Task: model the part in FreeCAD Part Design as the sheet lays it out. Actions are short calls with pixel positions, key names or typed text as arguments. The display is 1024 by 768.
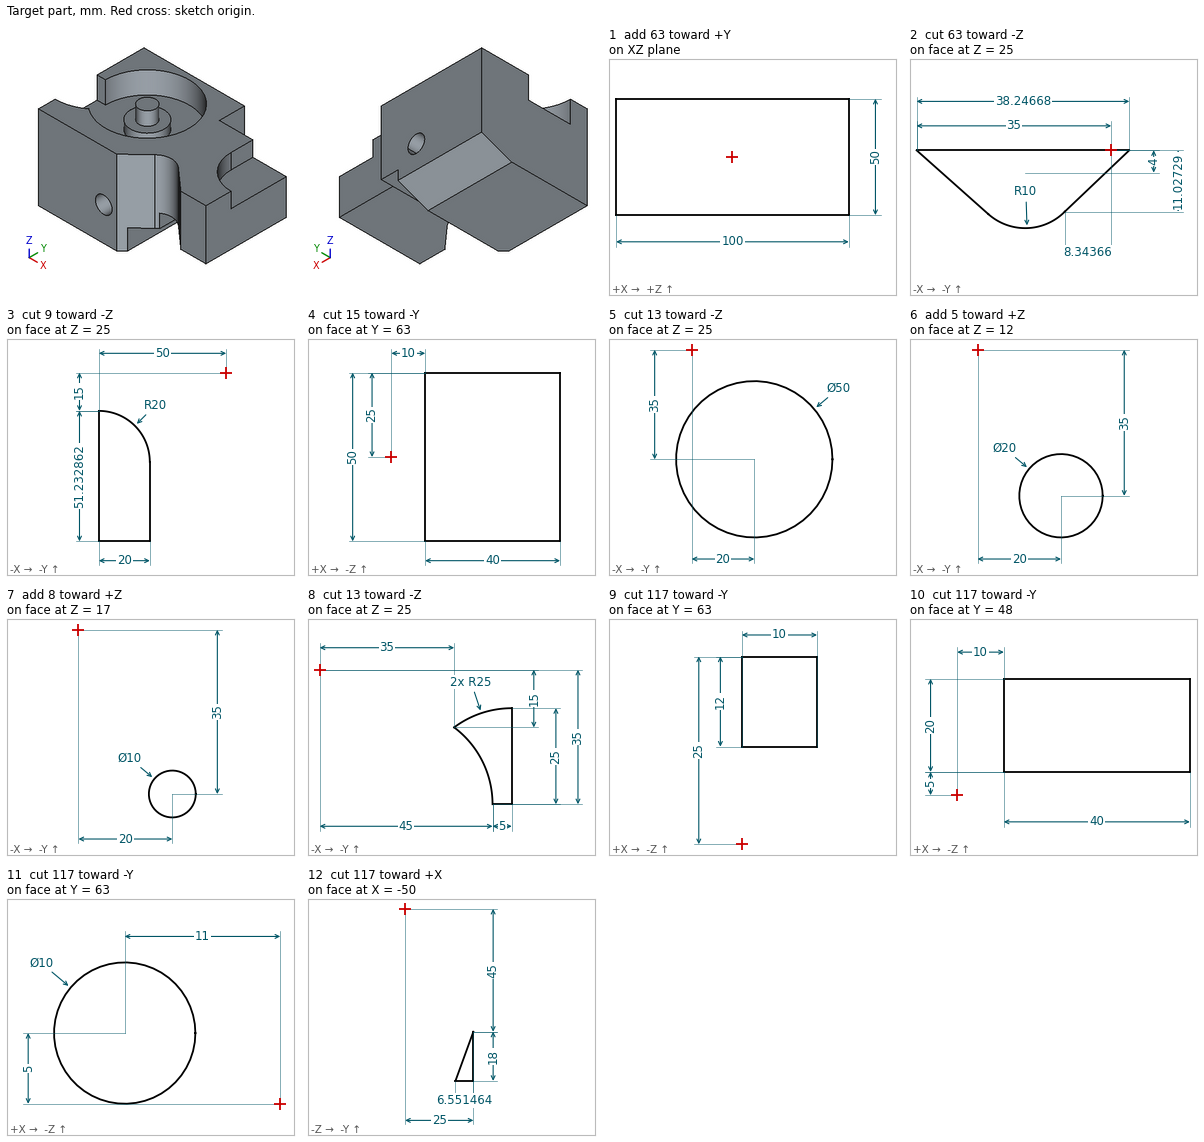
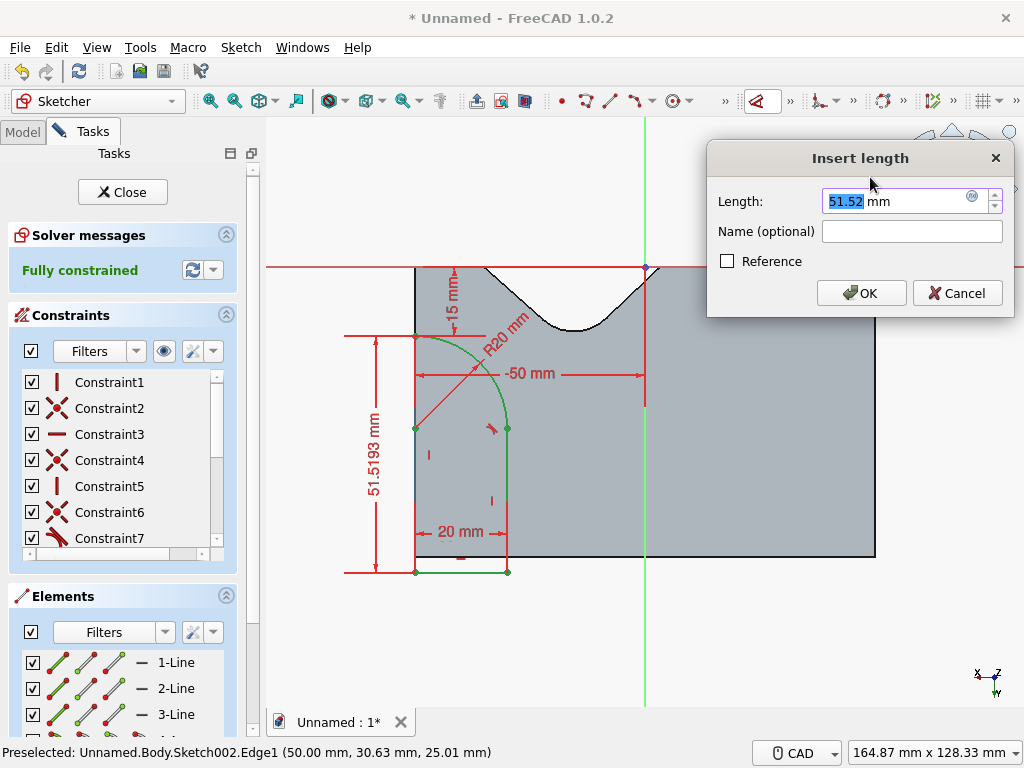
text(51.232862)
key(Return)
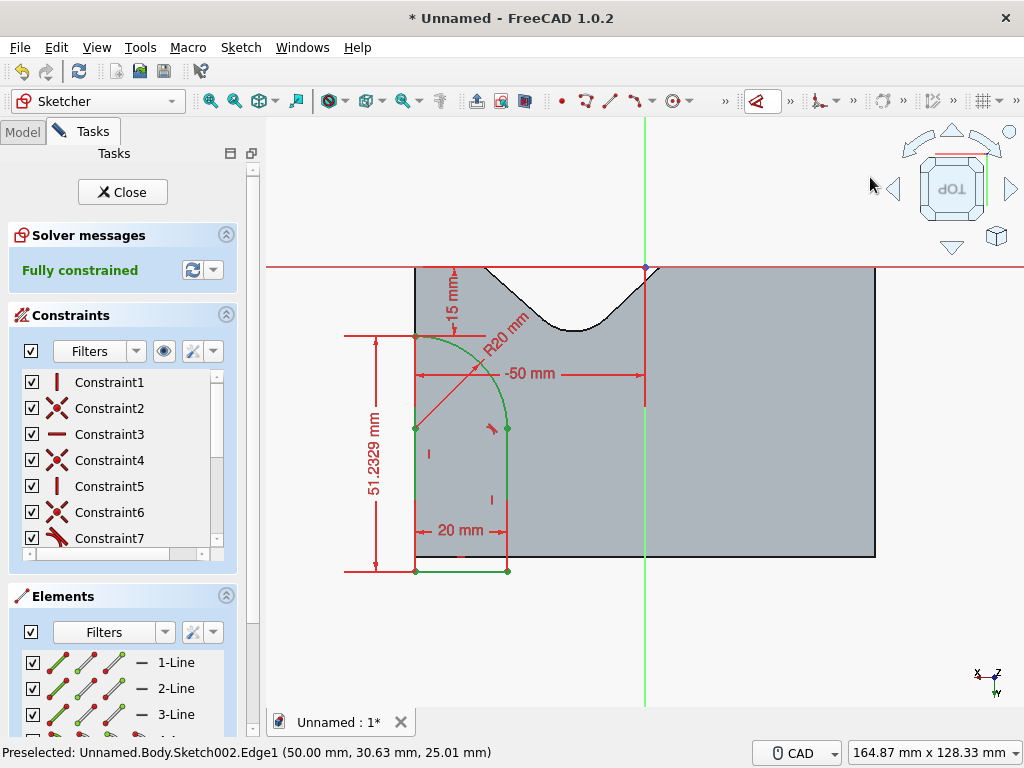
click(123, 192)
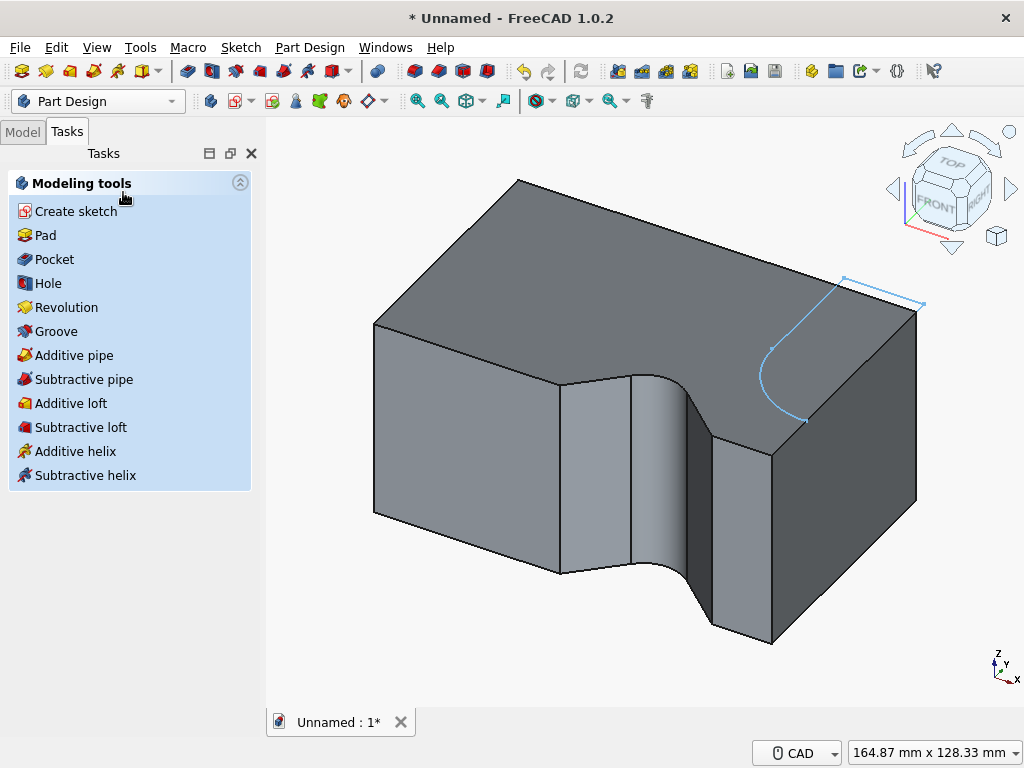
click(188, 72)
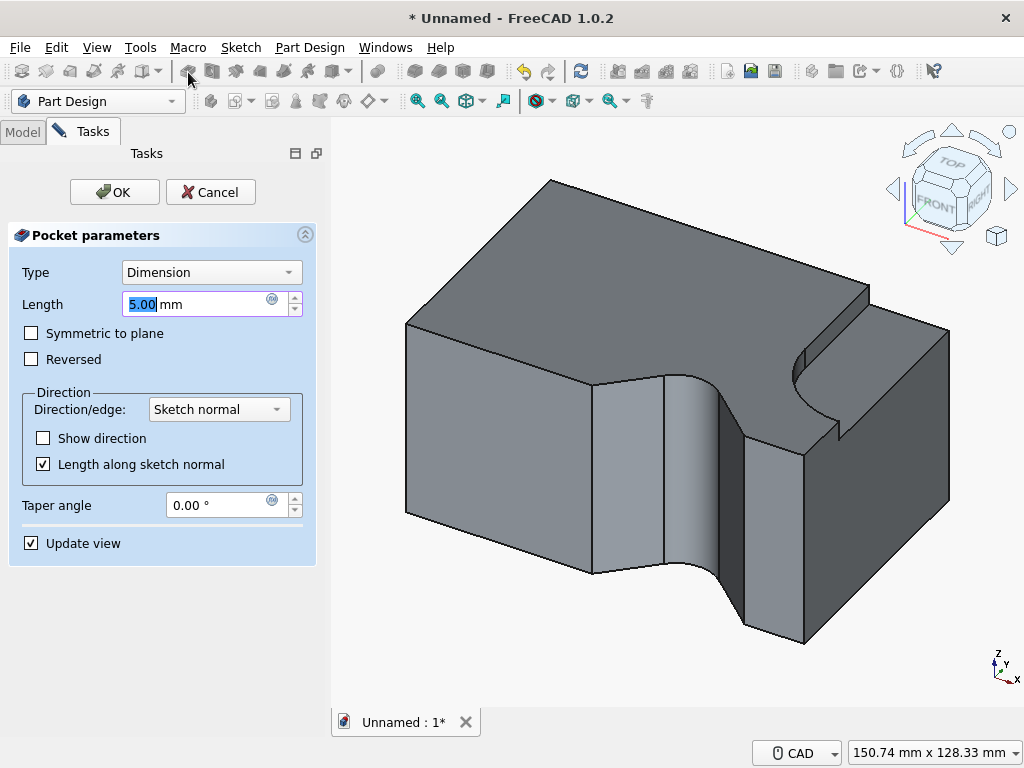
text(9)
key(Tab)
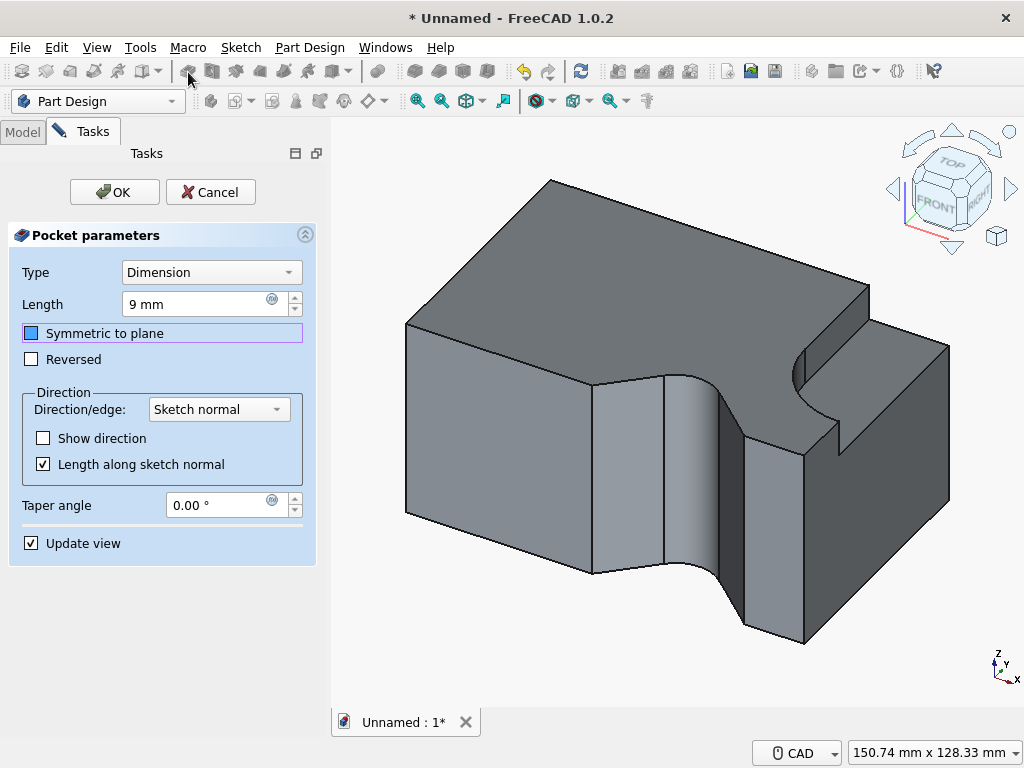
click(115, 192)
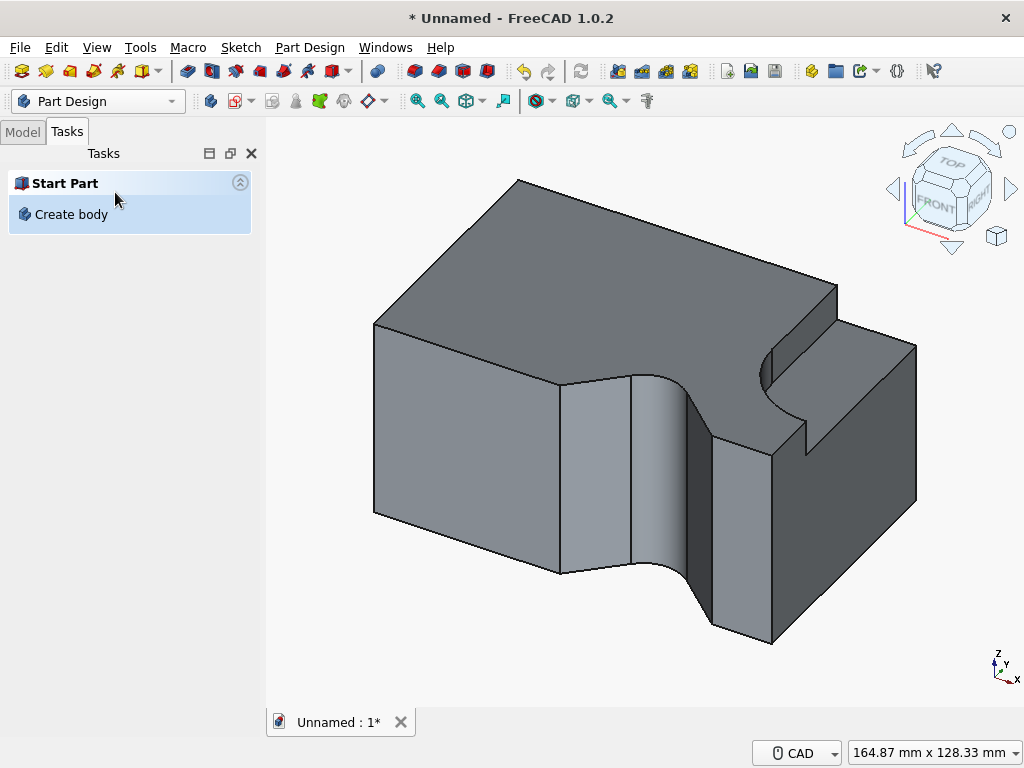
key(4)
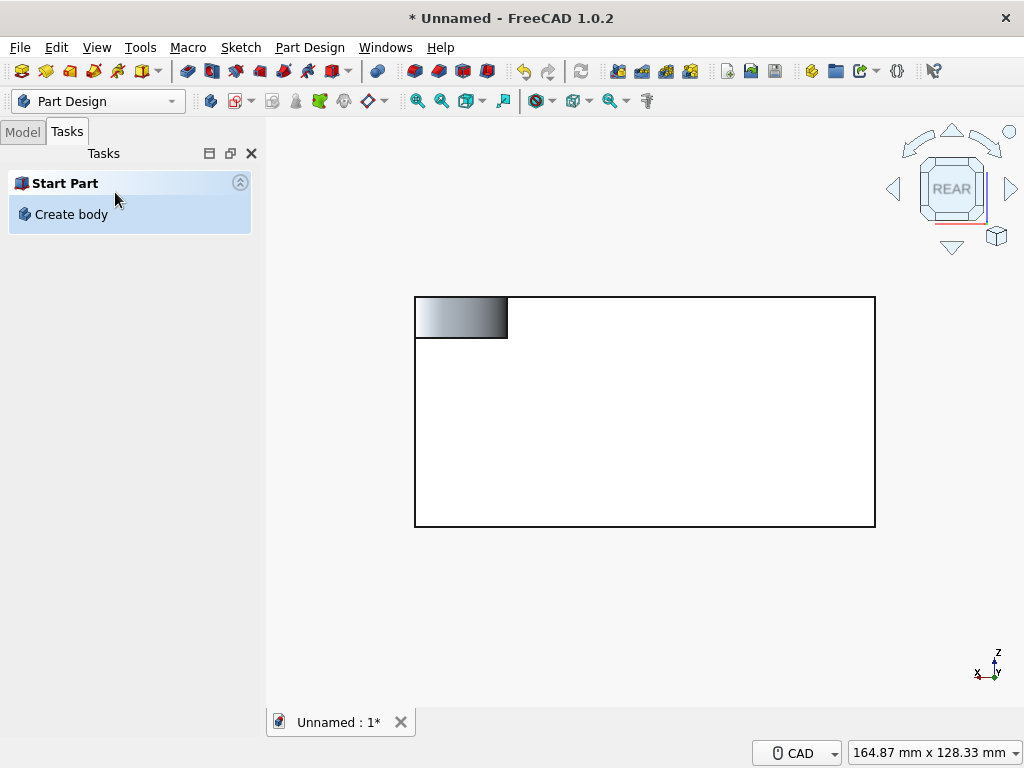
click(645, 411)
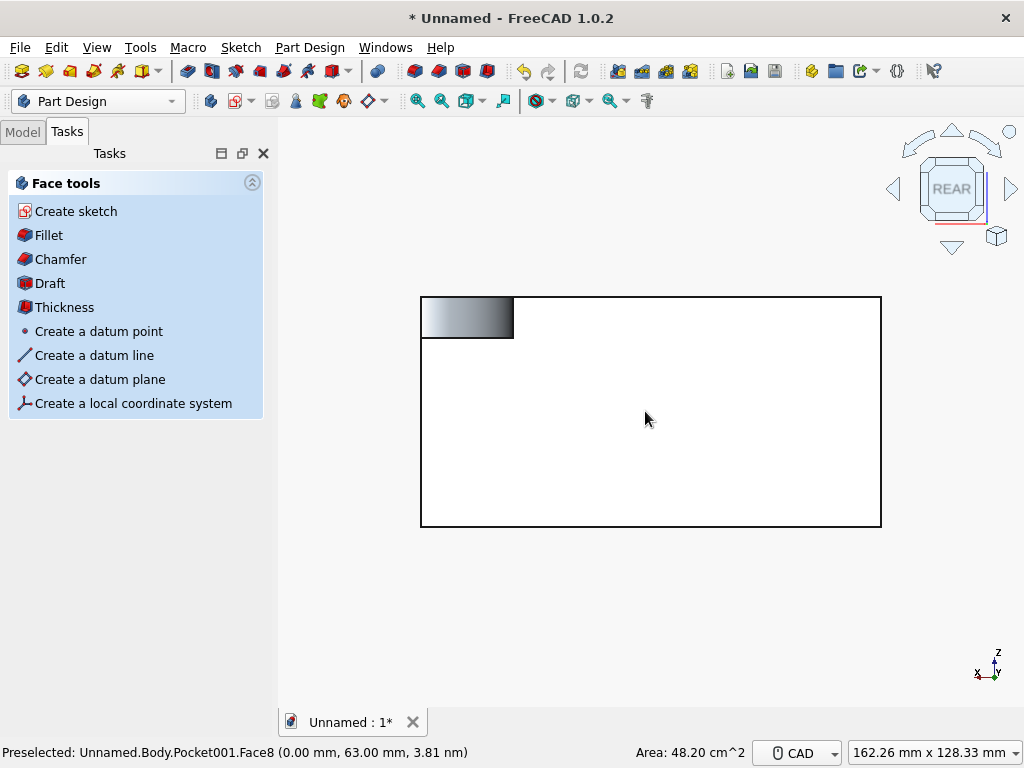
click(236, 102)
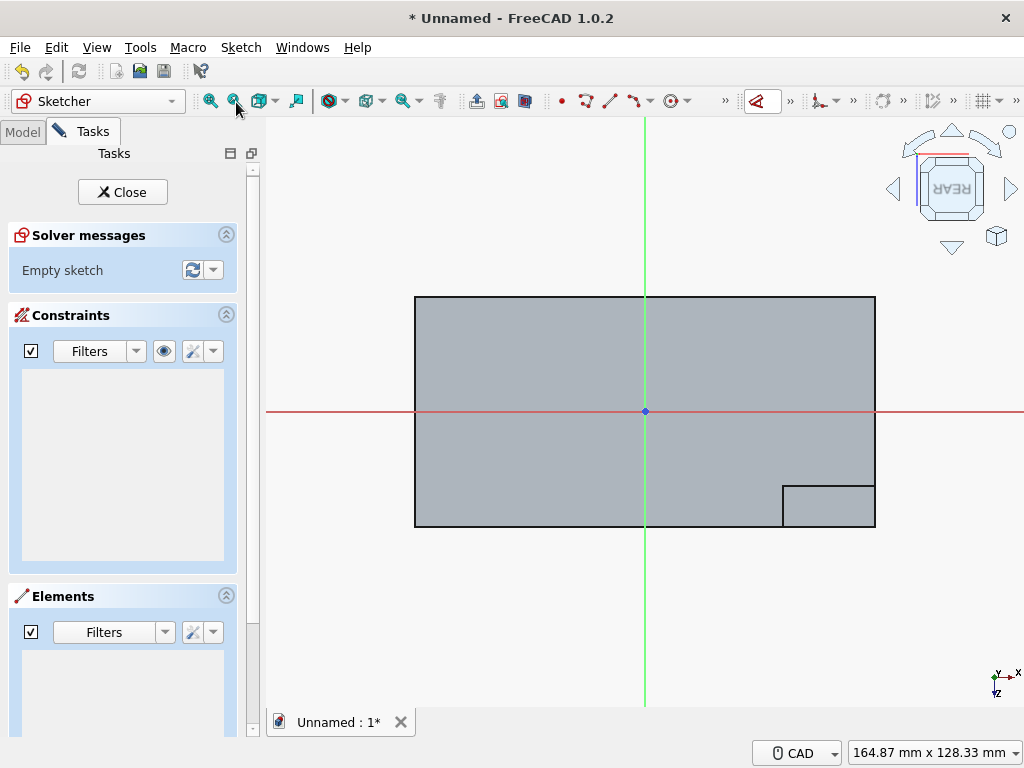
scroll(294, 412, down, 1)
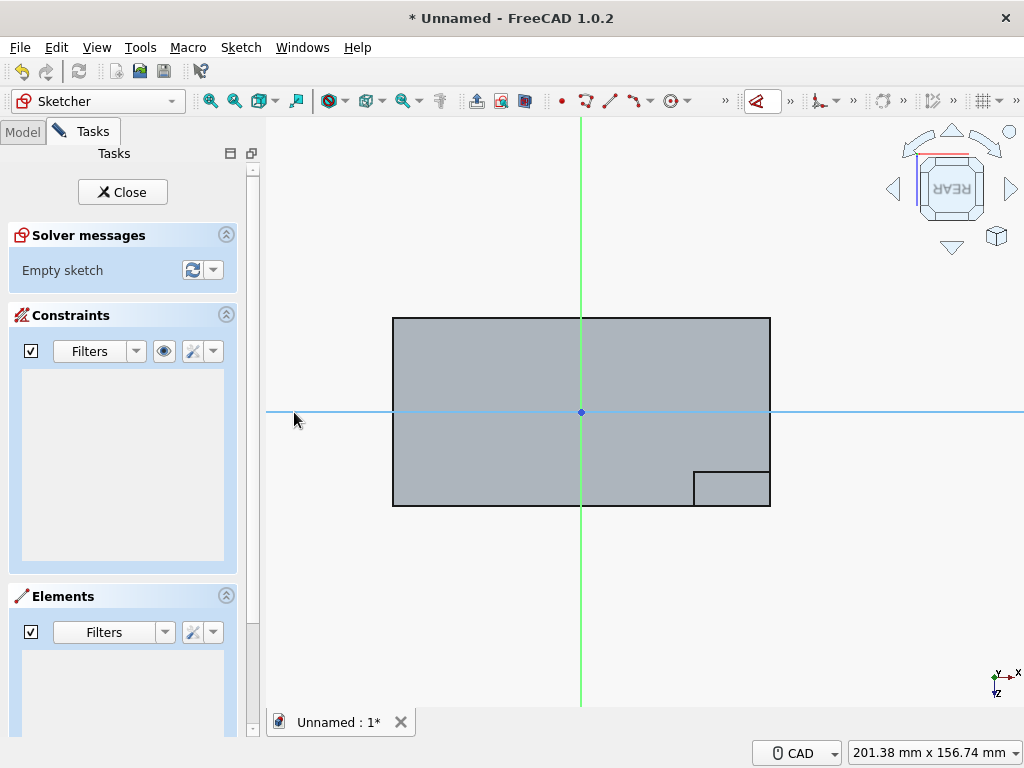
scroll(796, 412, up, 3)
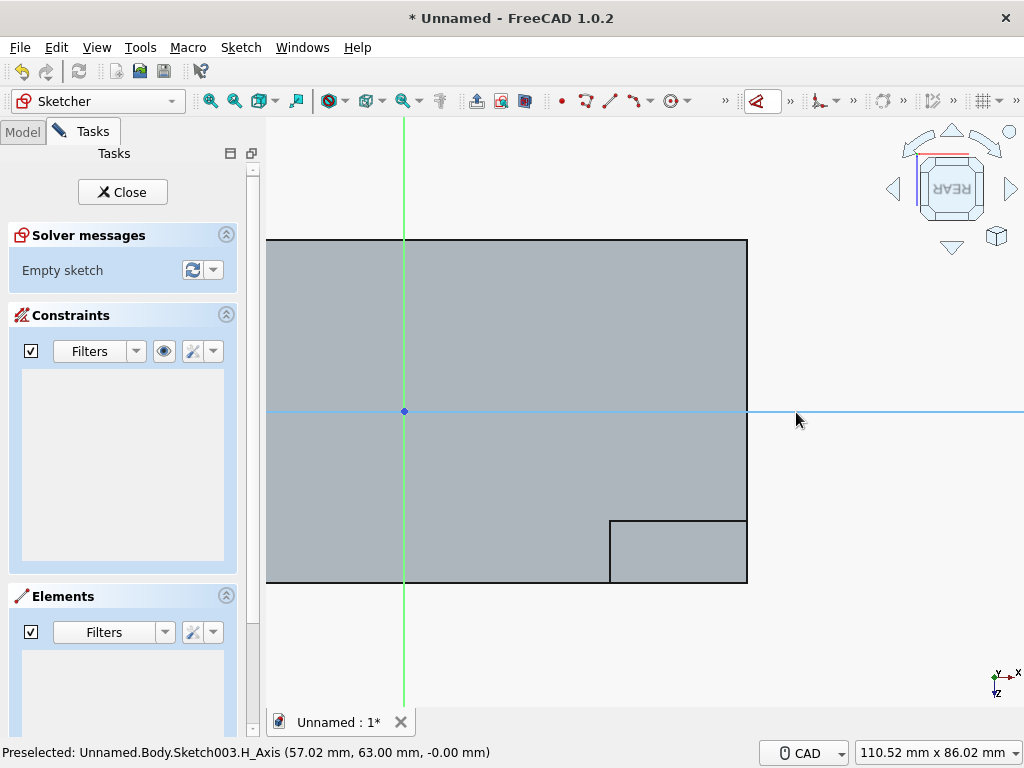
key(g)
key(r)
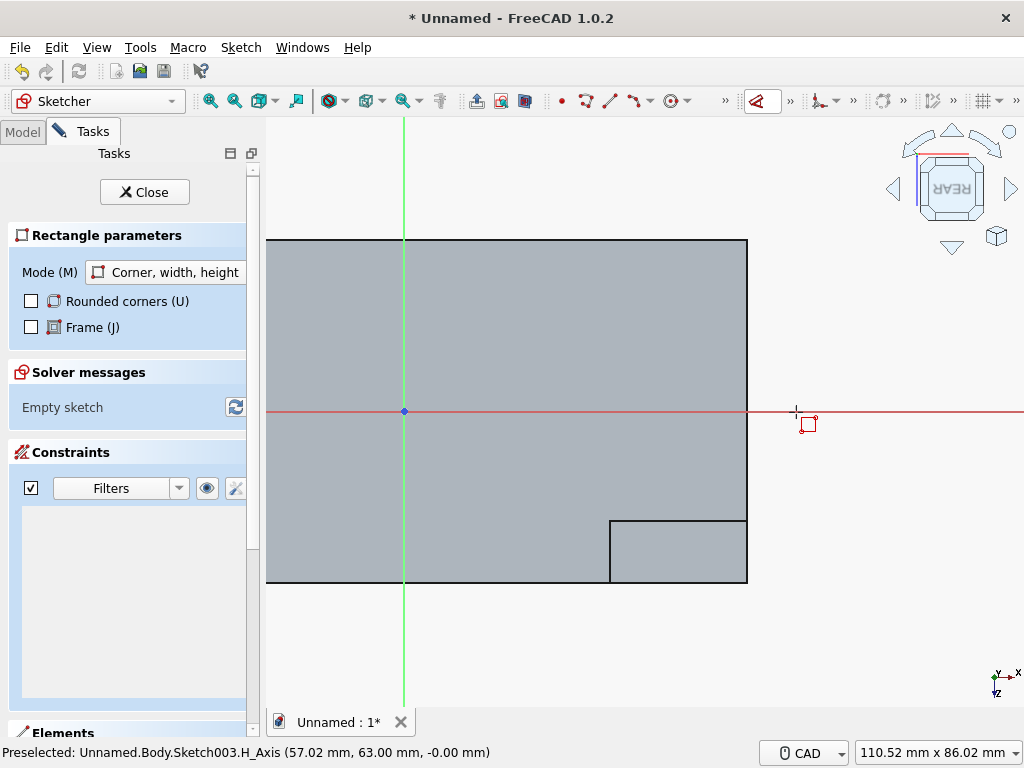
click(473, 240)
click(747, 583)
key(Escape)